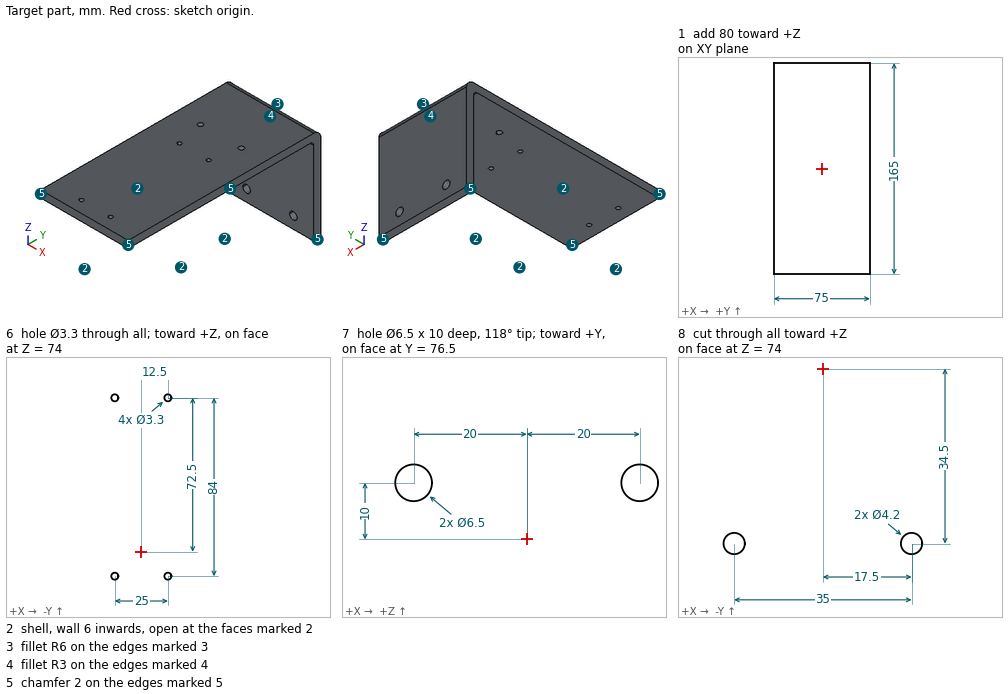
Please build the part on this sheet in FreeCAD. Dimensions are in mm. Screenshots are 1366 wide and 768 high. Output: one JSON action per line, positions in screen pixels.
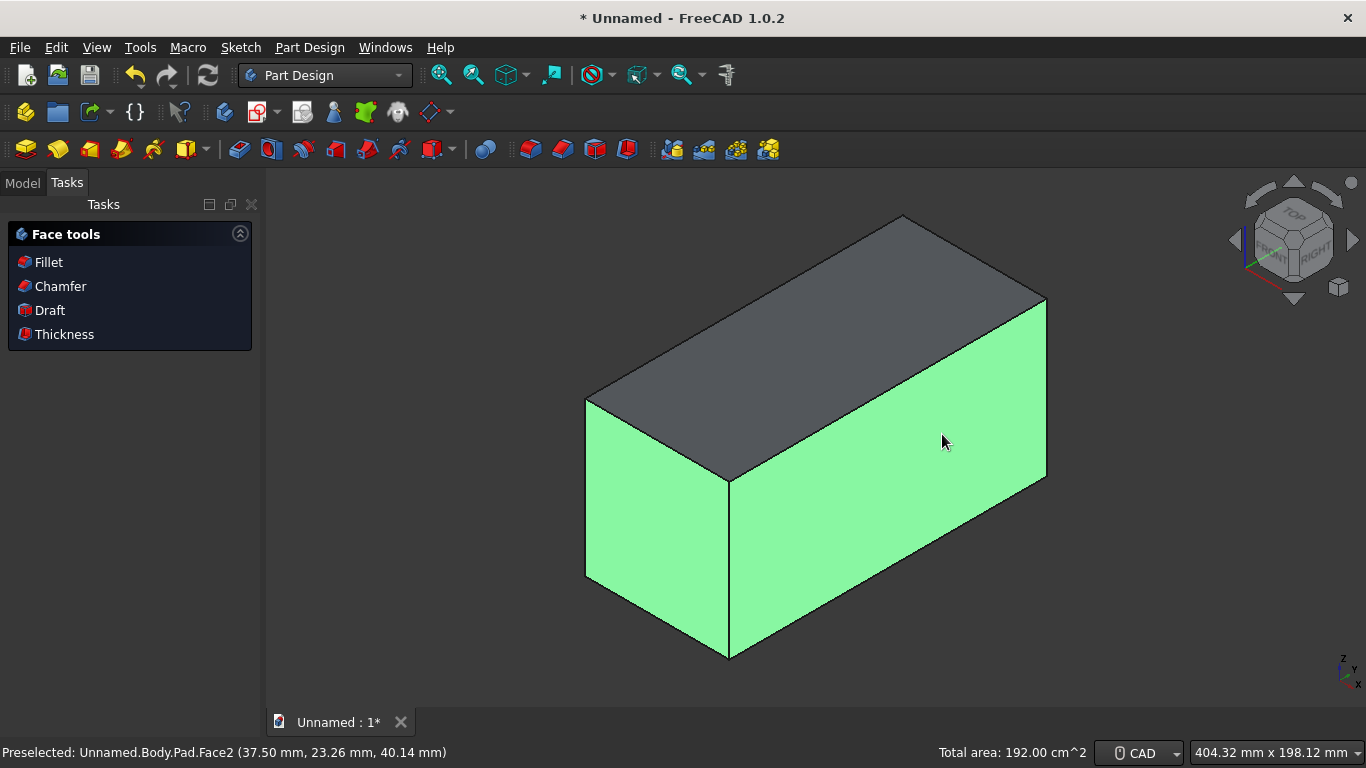
{"action": "key", "text": "2"}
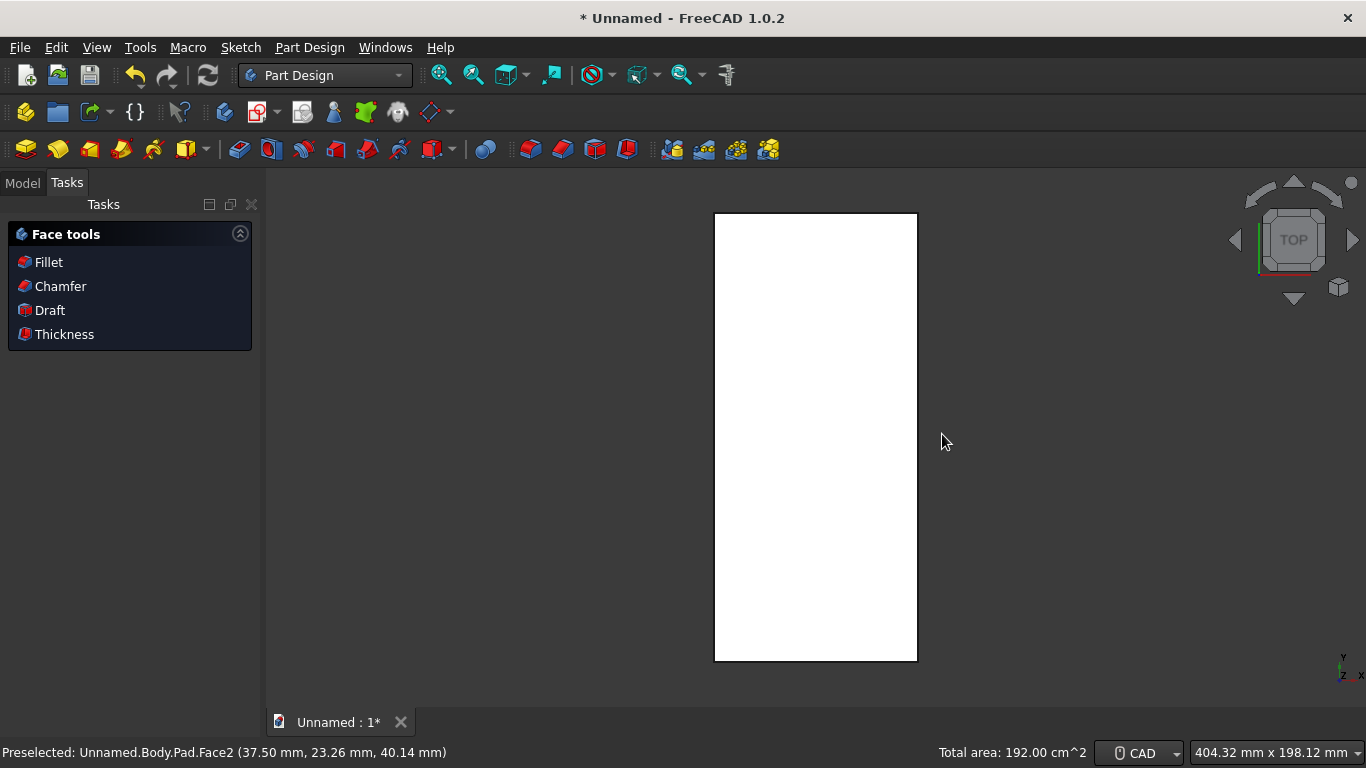
{"action": "key", "text": "1"}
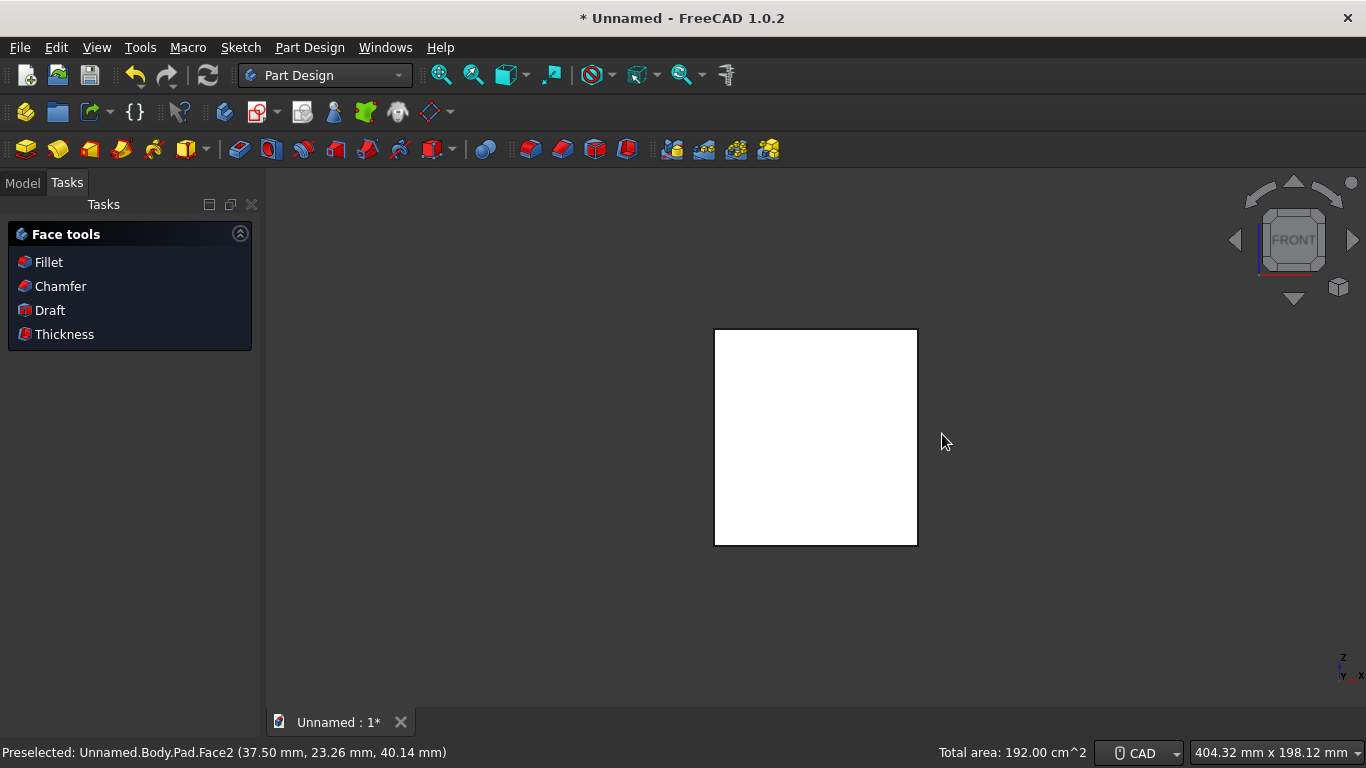
{"action": "left_click", "coordinate": [442, 76]}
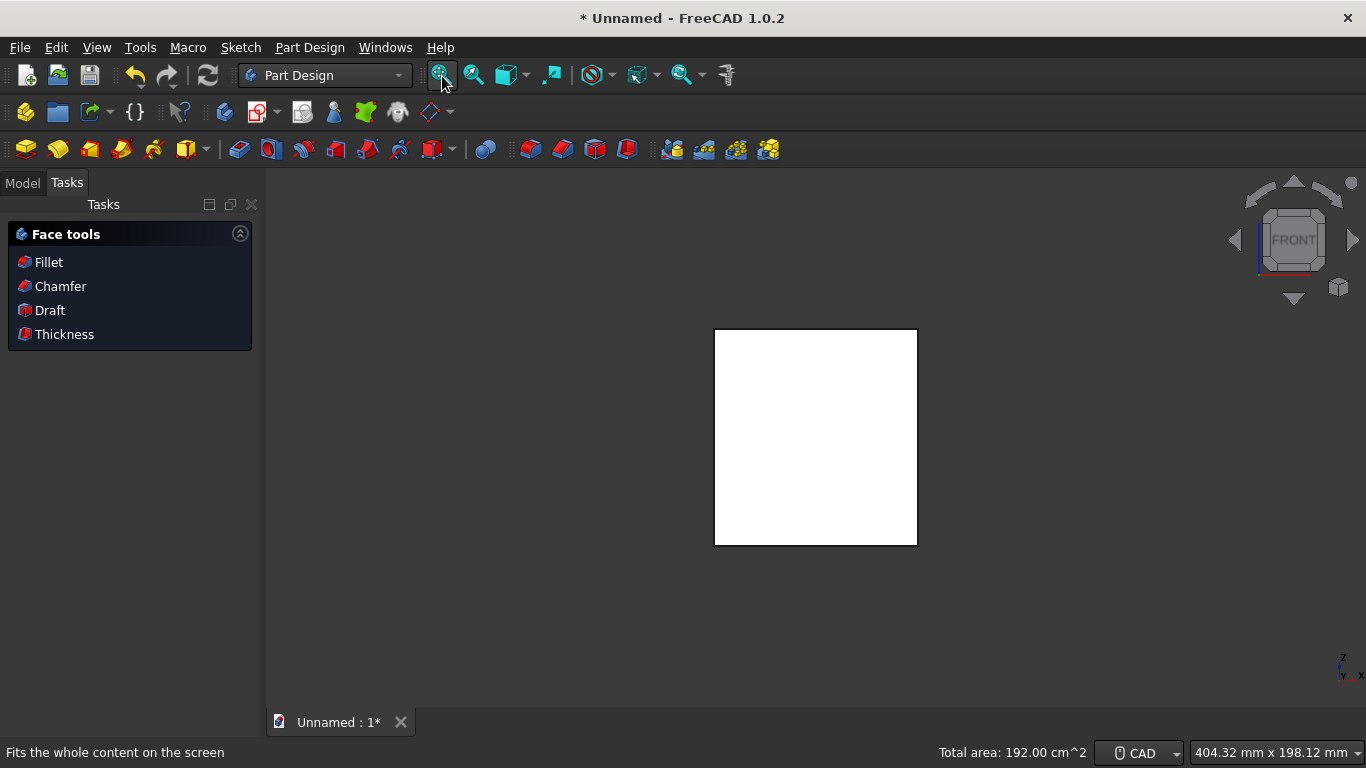
{"action": "key", "text": "3"}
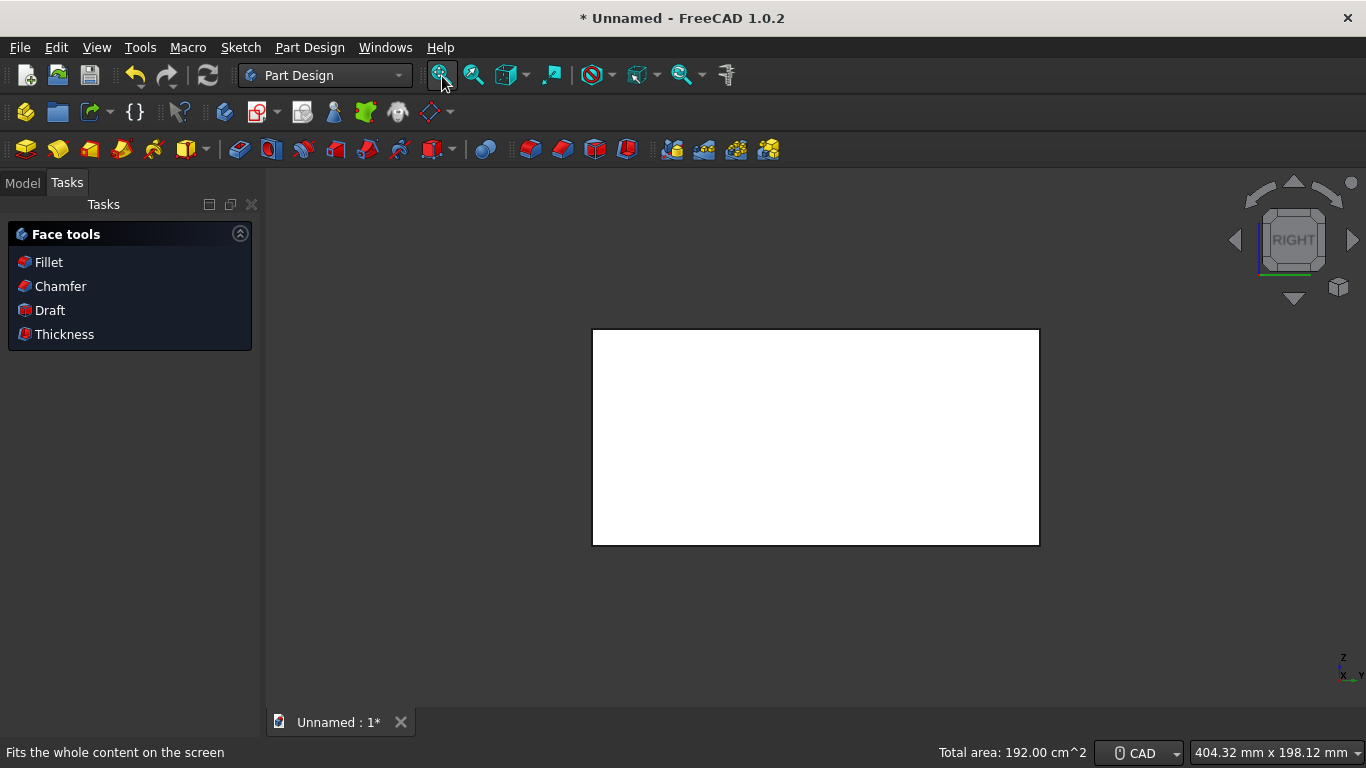
{"action": "left_click", "coordinate": [442, 76]}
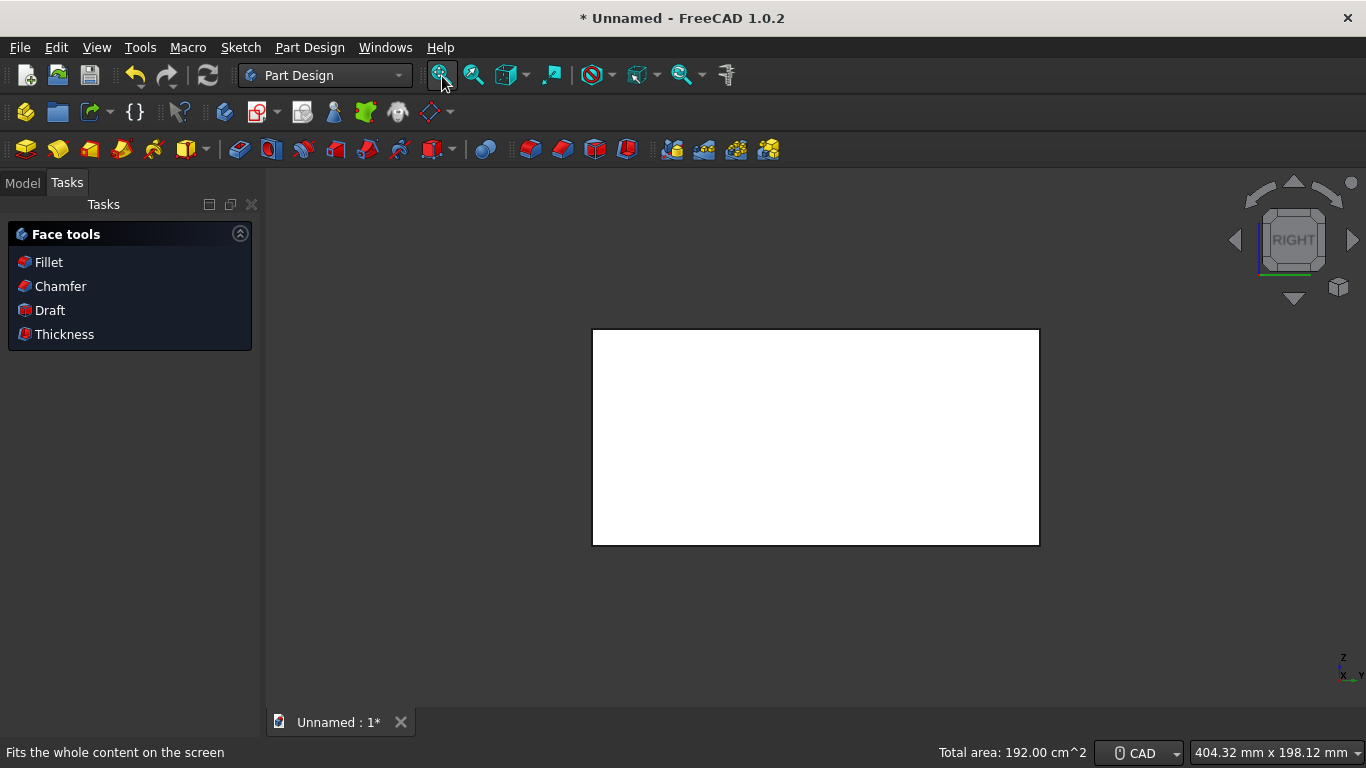
{"action": "key", "text": "5"}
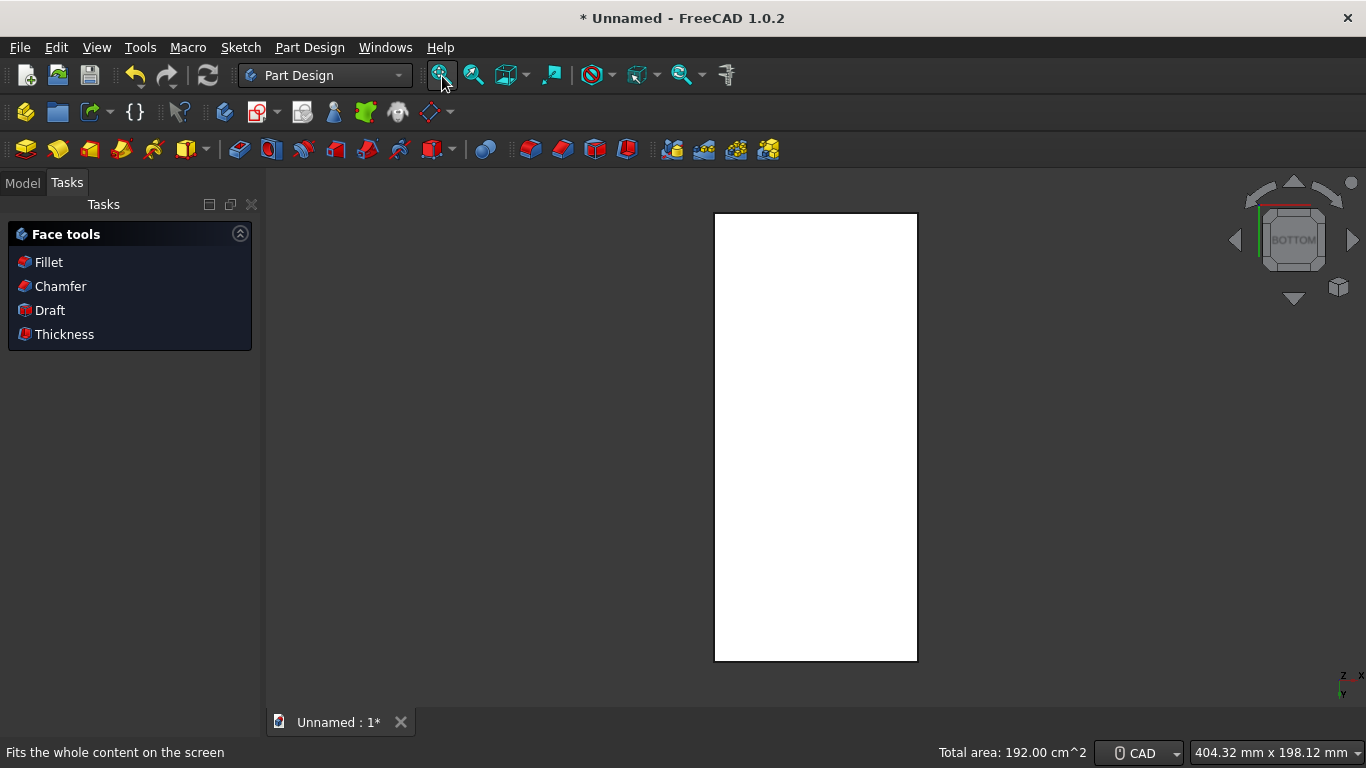
{"action": "left_click", "coordinate": [816, 501], "text": "ctrl"}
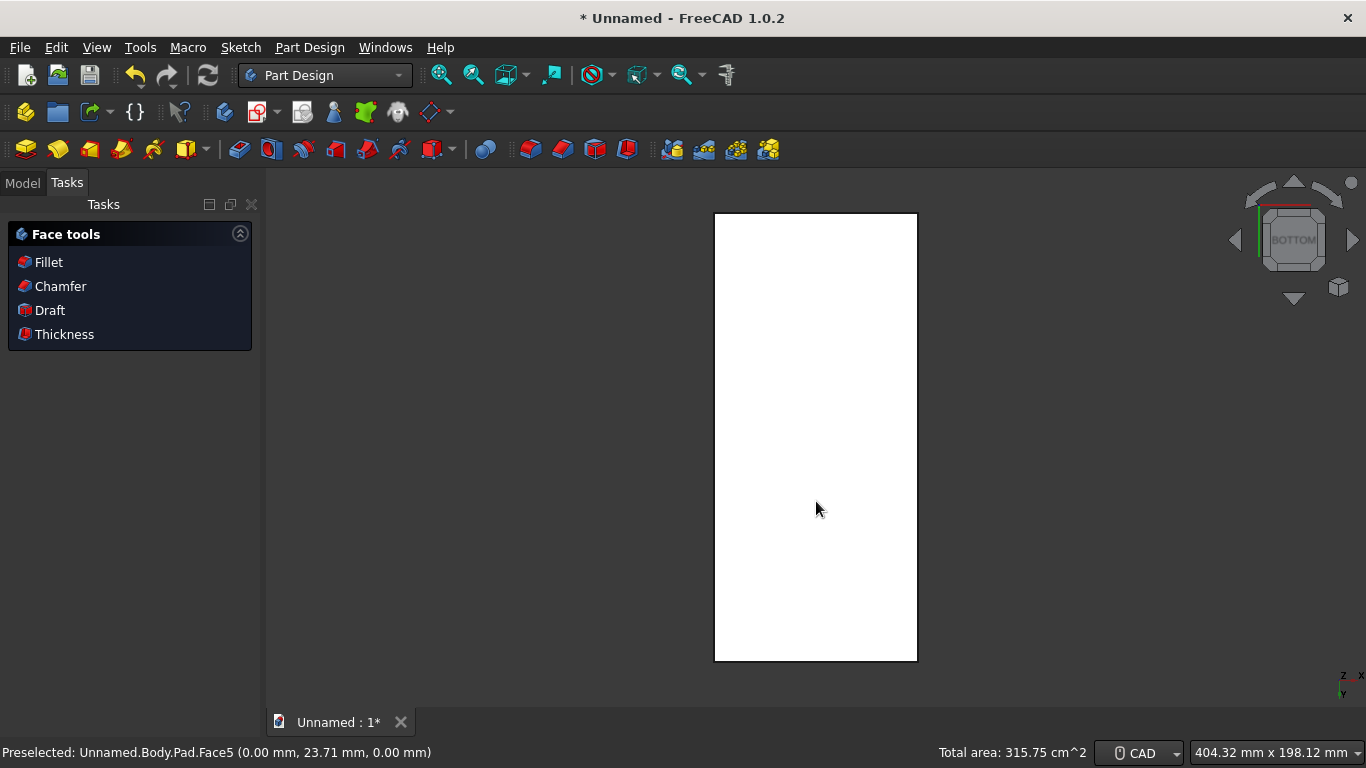
{"action": "key", "text": "4"}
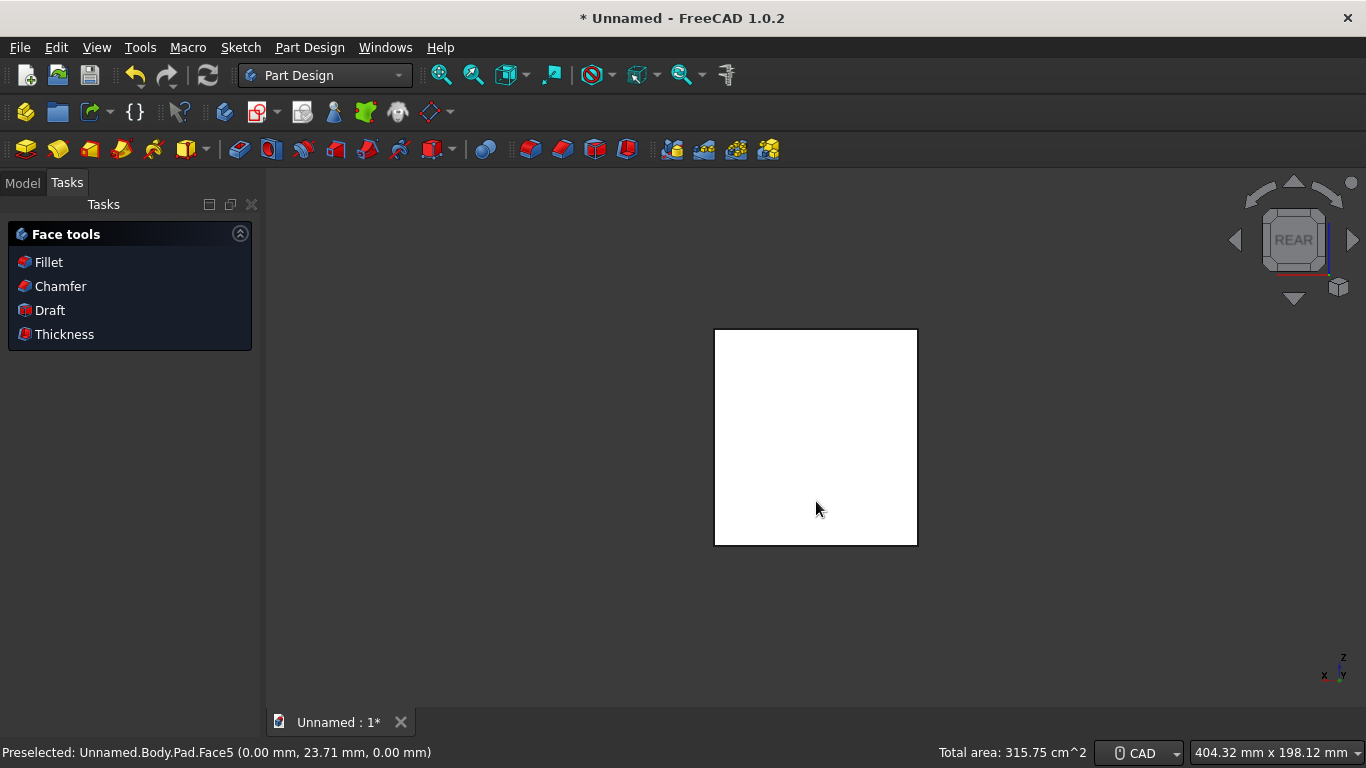
{"action": "left_click", "coordinate": [442, 76]}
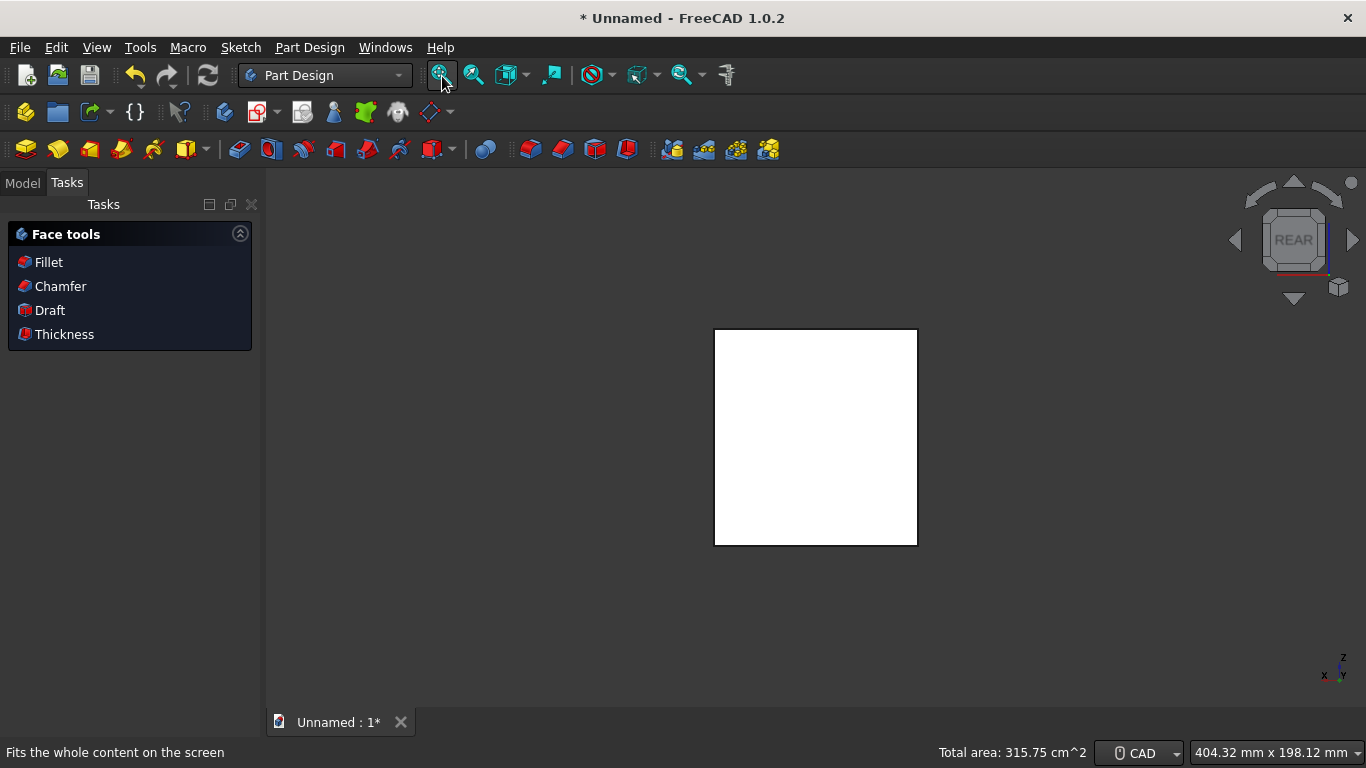
{"action": "key", "text": "6"}